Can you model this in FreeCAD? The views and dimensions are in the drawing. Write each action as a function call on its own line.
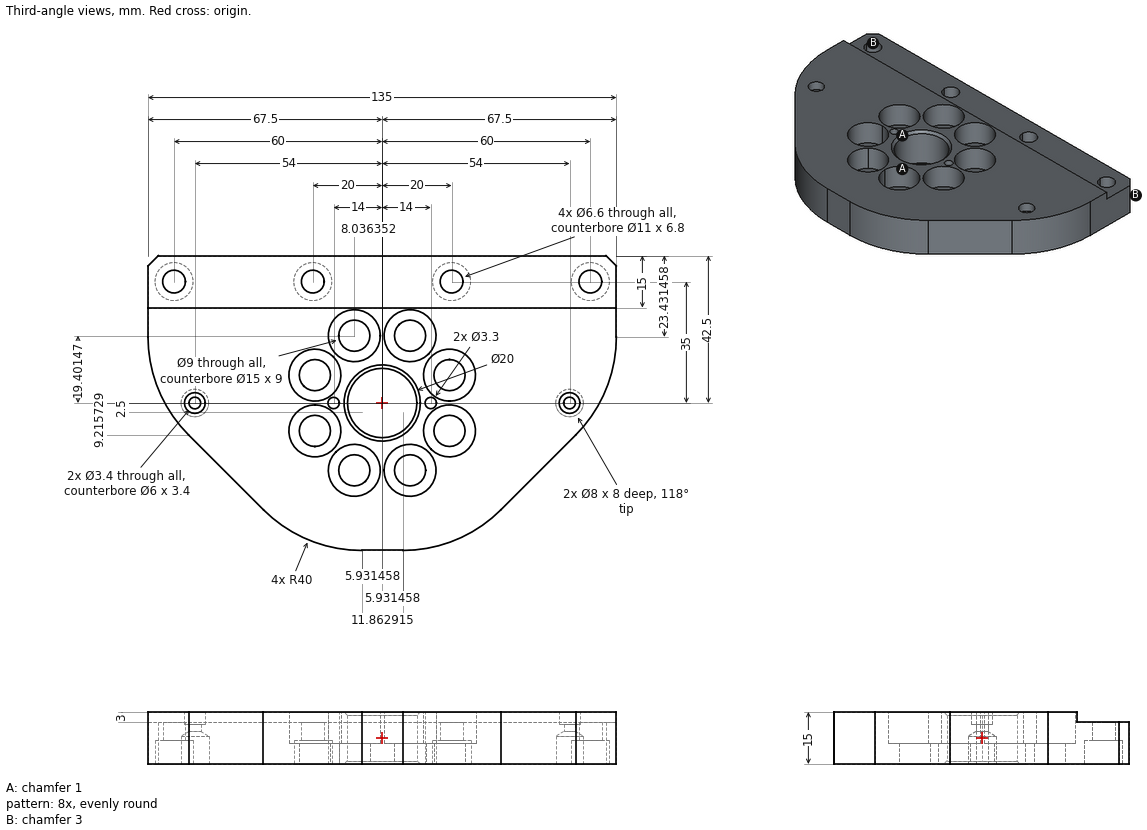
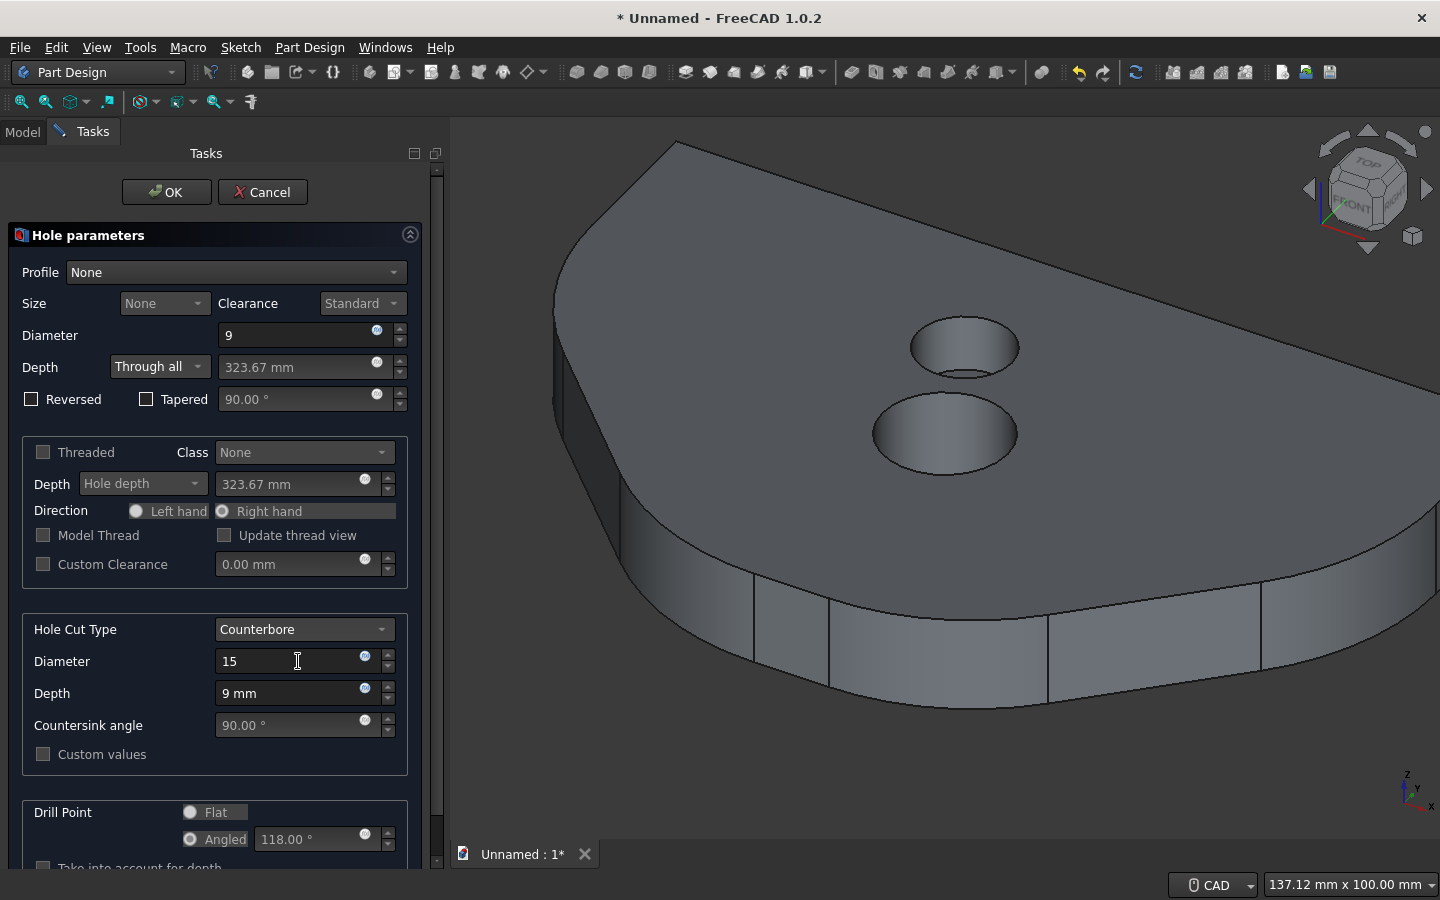
click(167, 192)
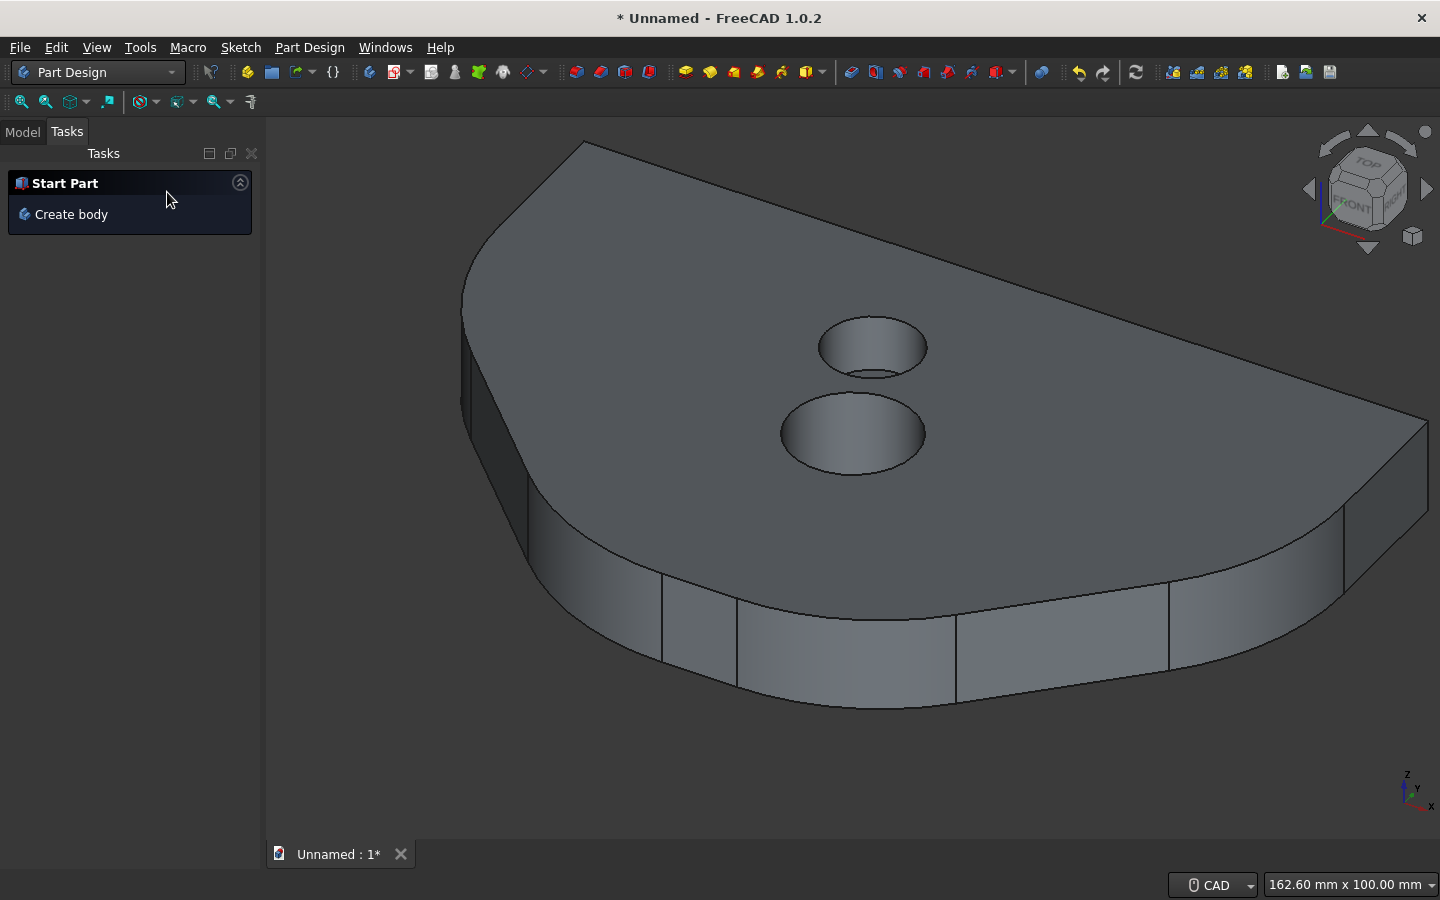
click(790, 412)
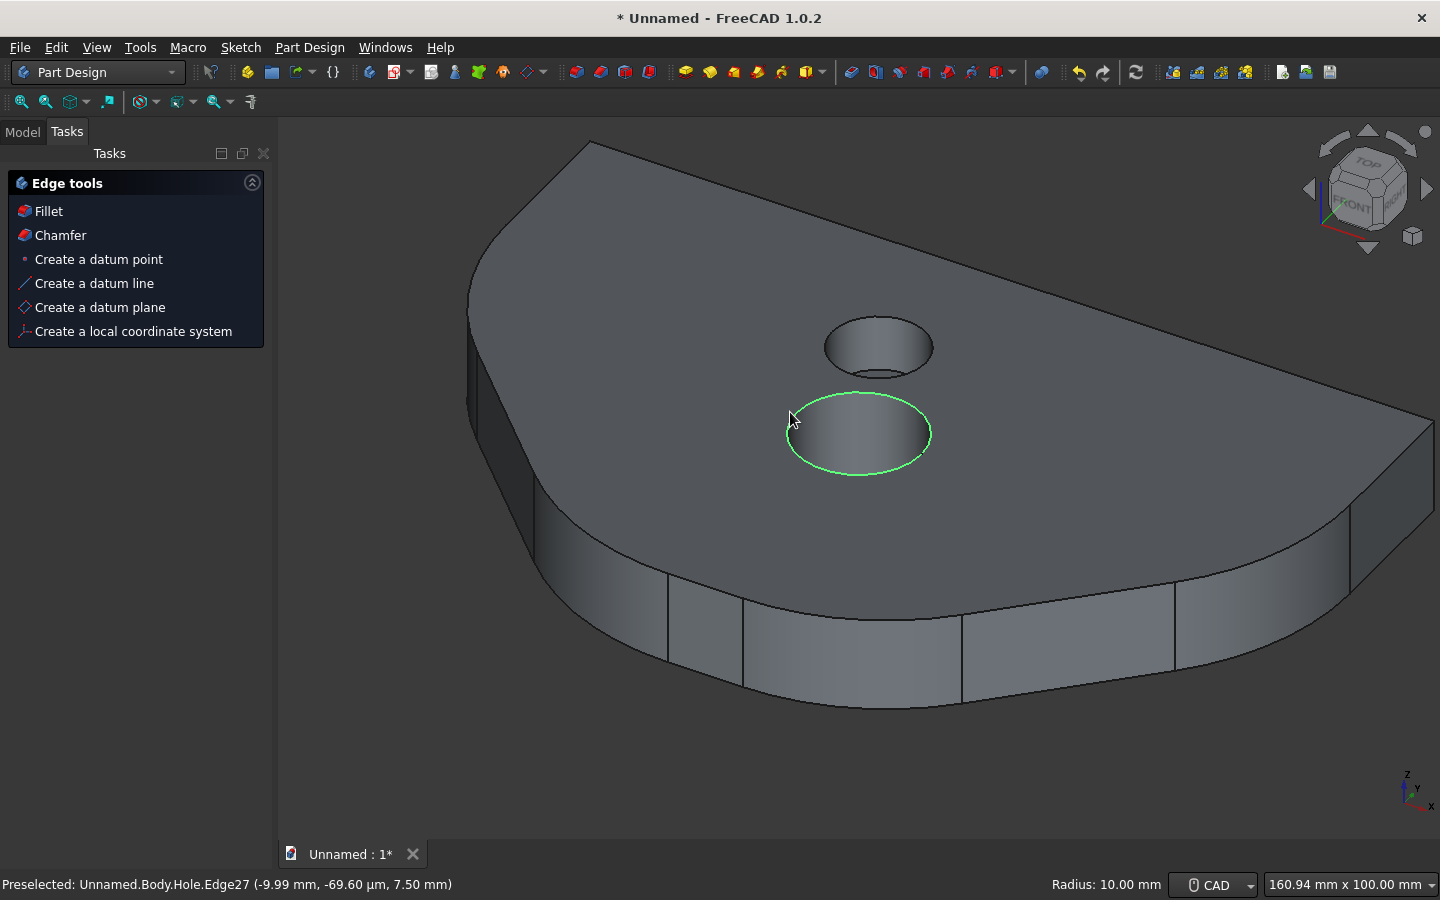
key(0)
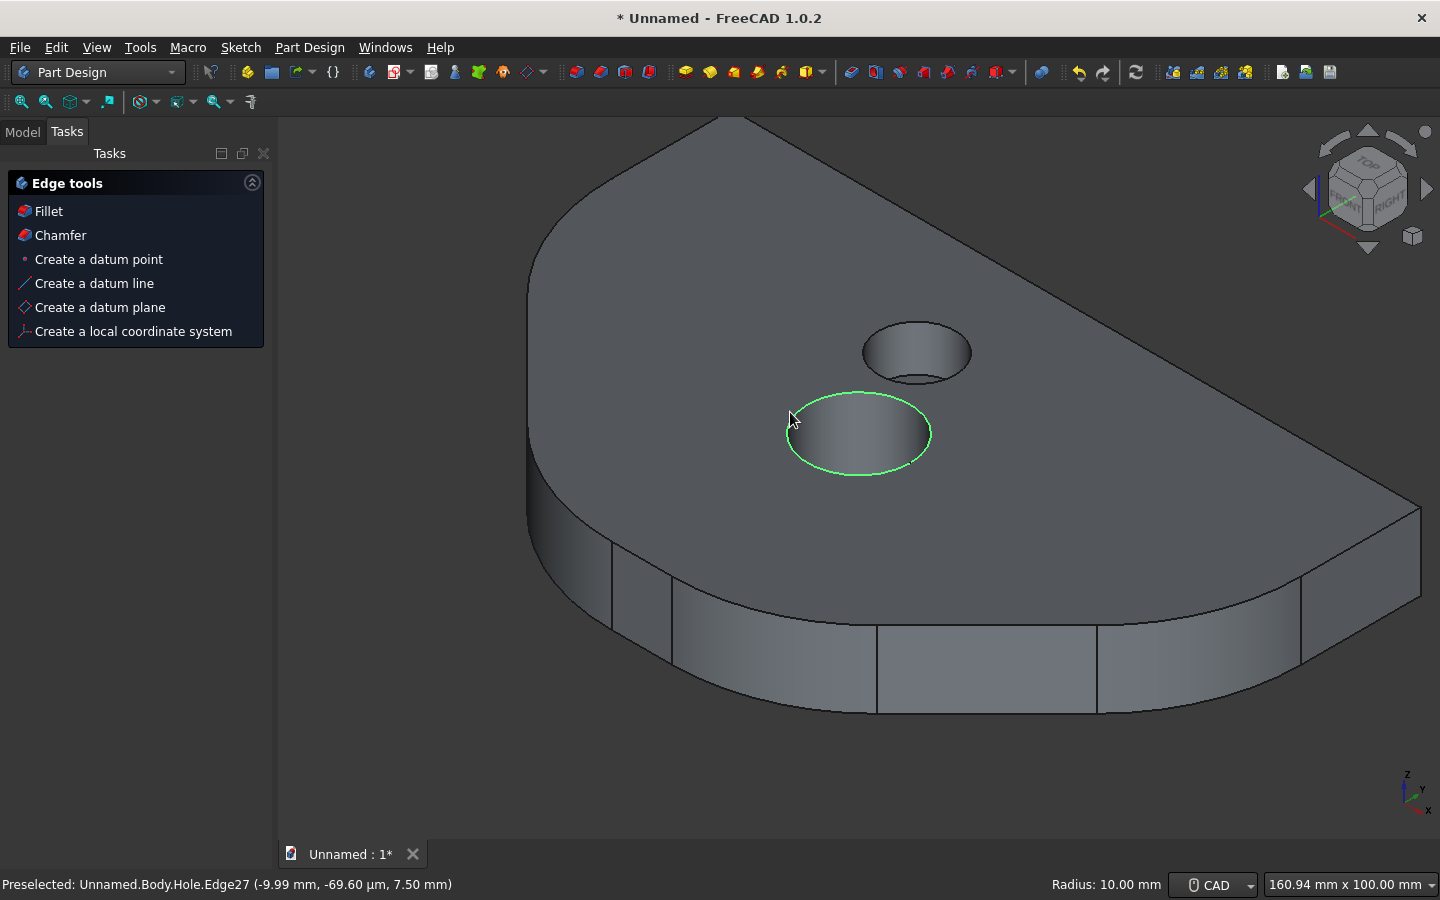
click(22, 102)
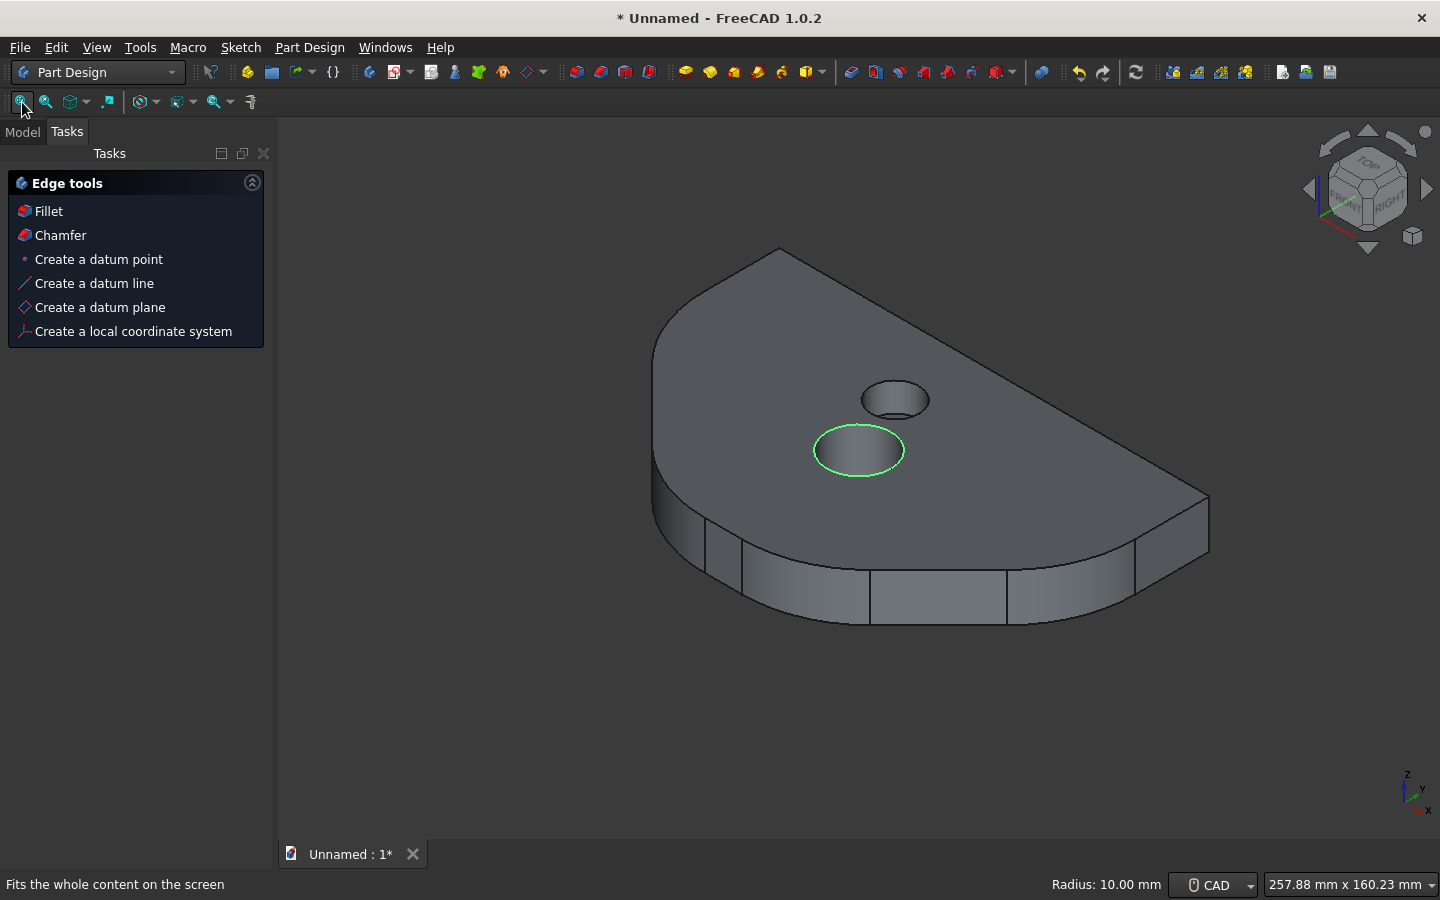
key(2)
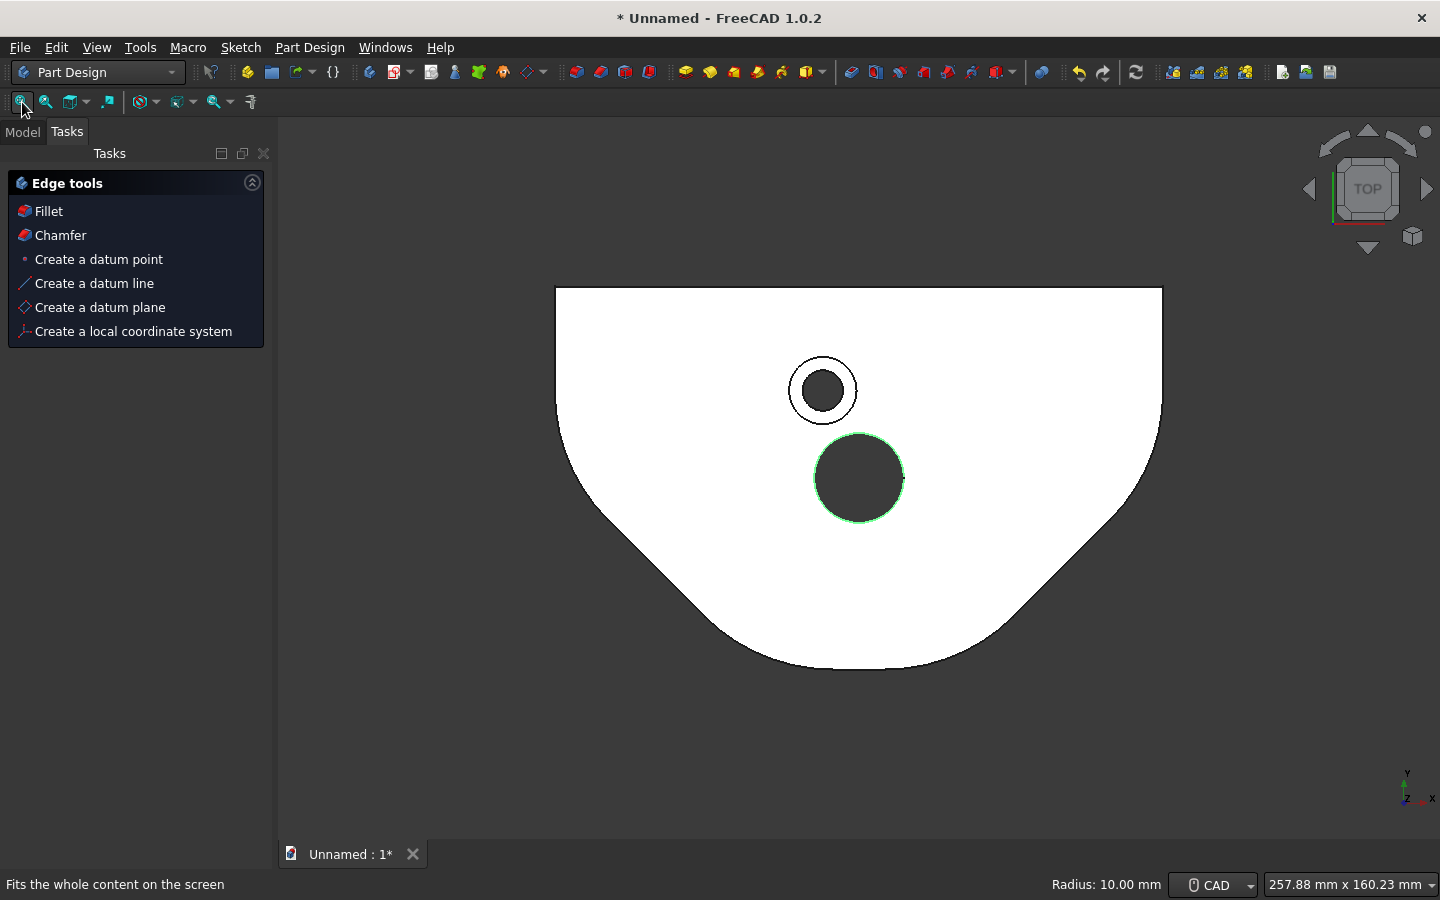
key(1)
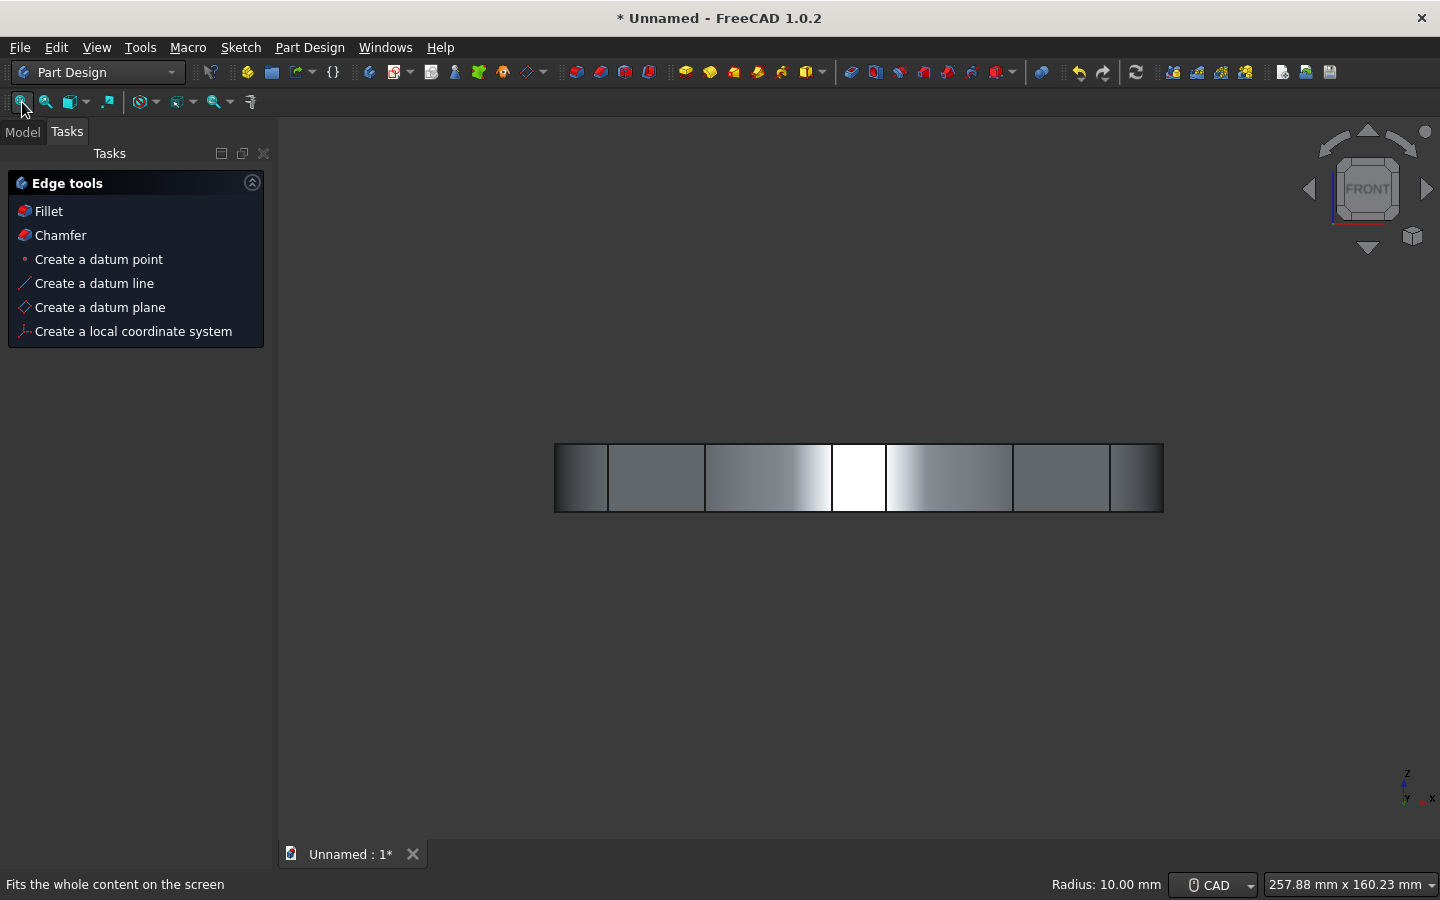
key(3)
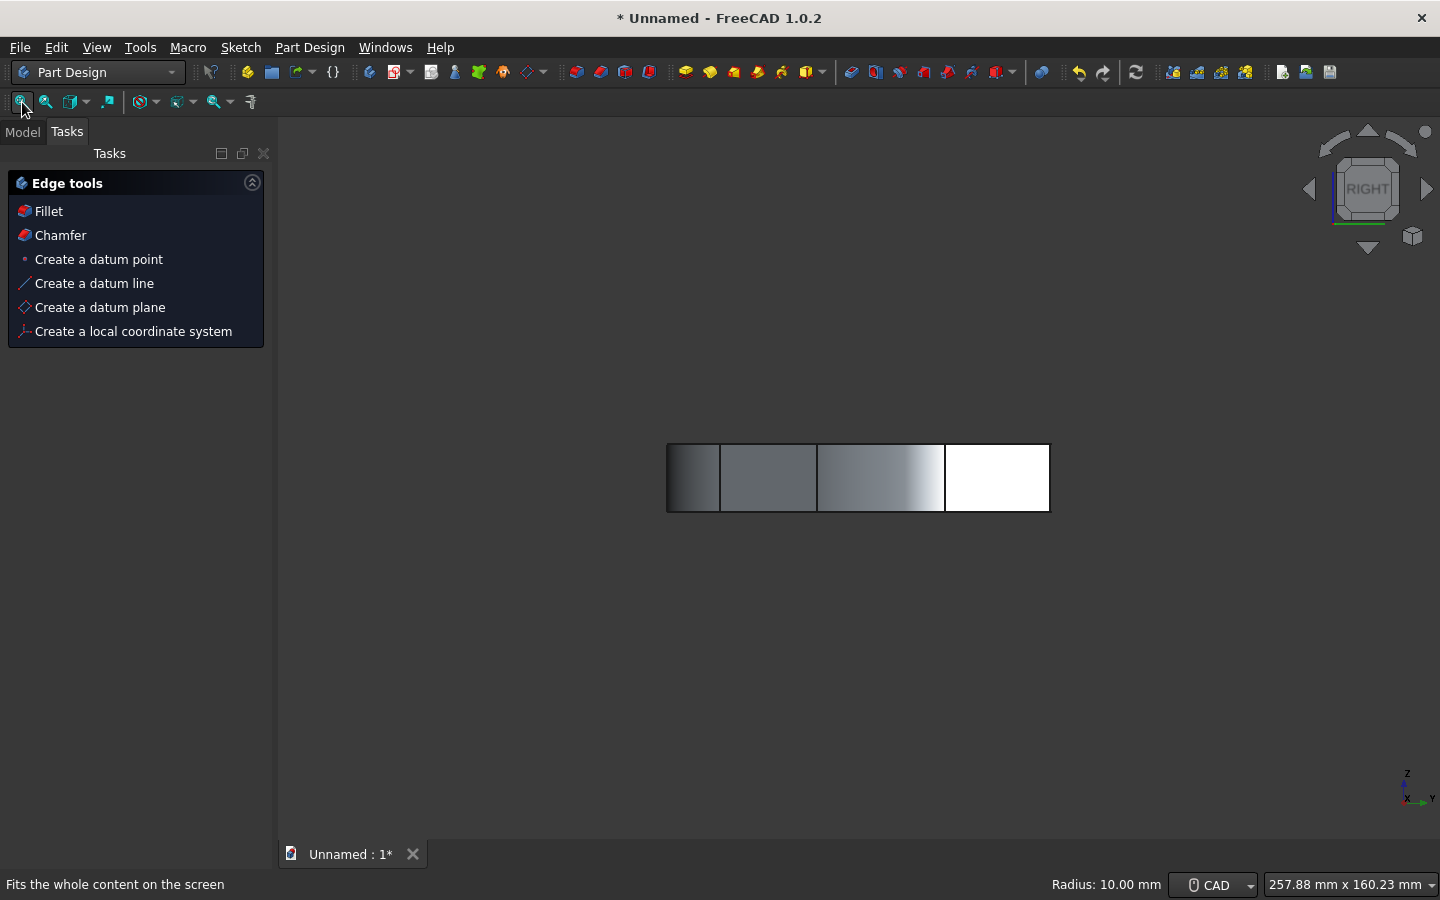
click(22, 102)